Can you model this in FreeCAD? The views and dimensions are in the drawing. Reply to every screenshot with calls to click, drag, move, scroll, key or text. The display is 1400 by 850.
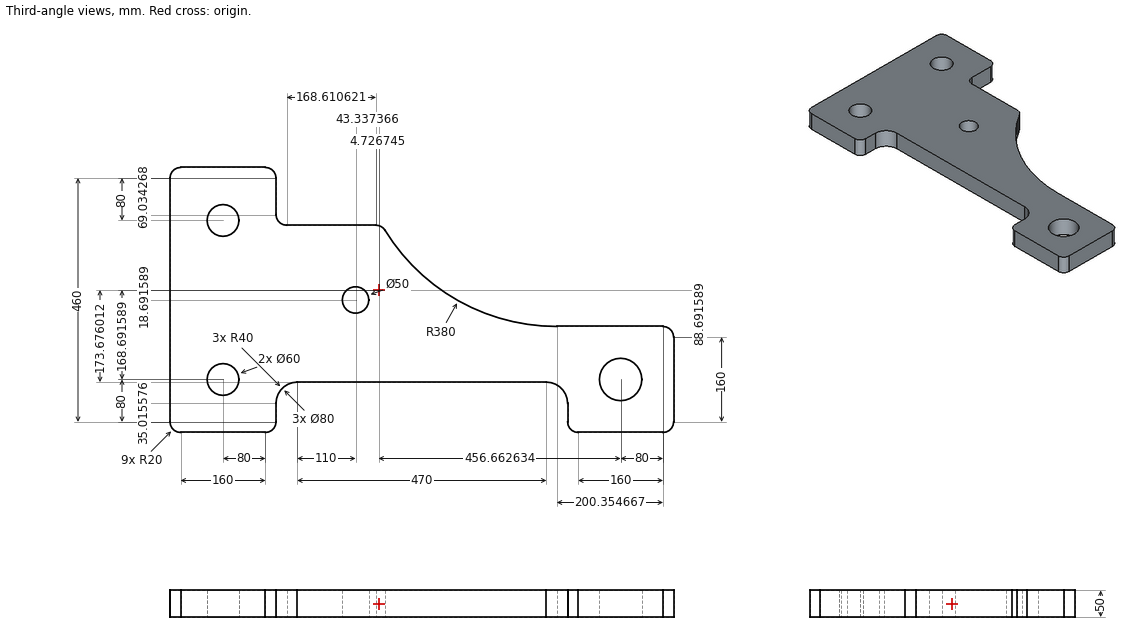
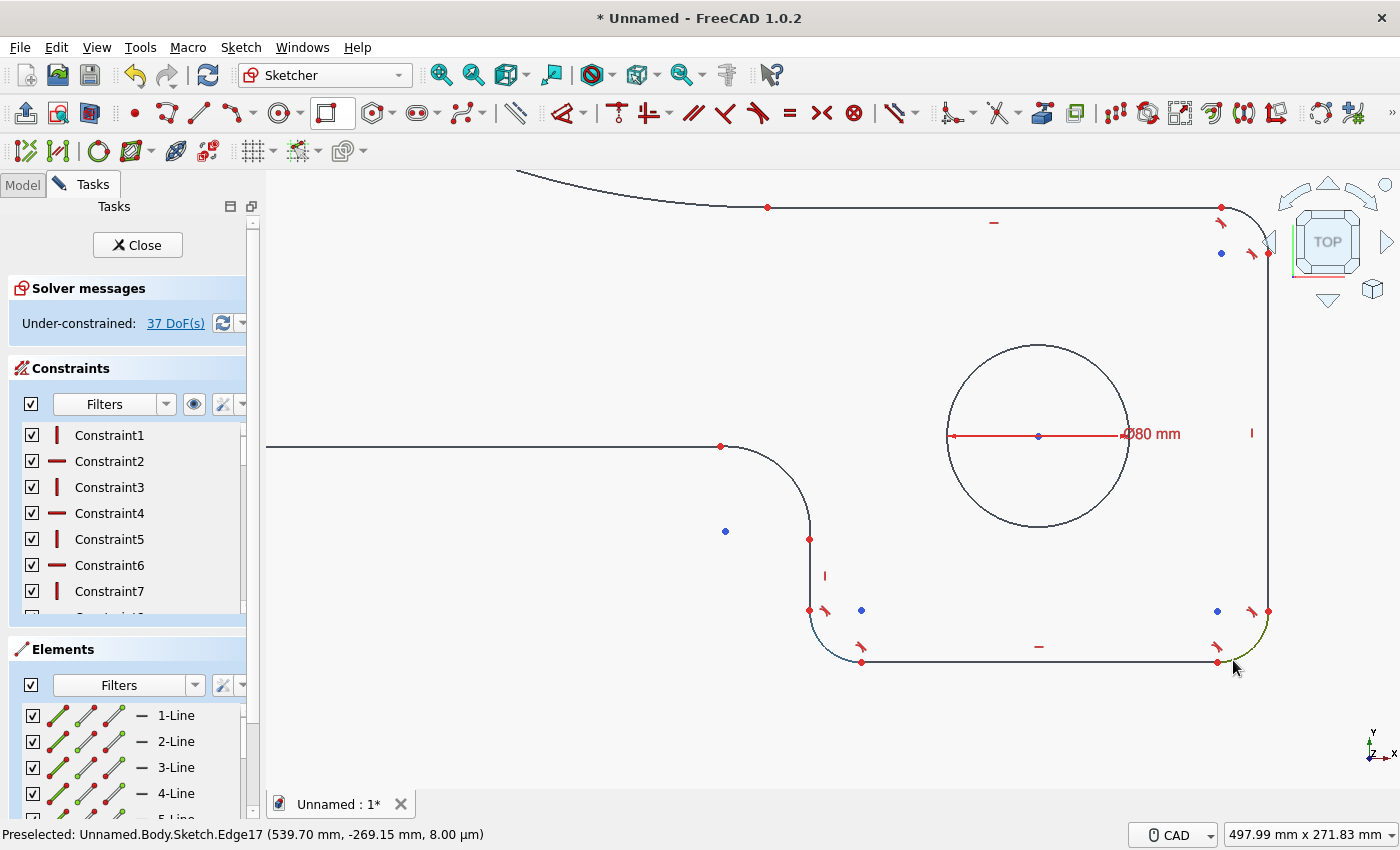
scroll(1014, 647, down, 6)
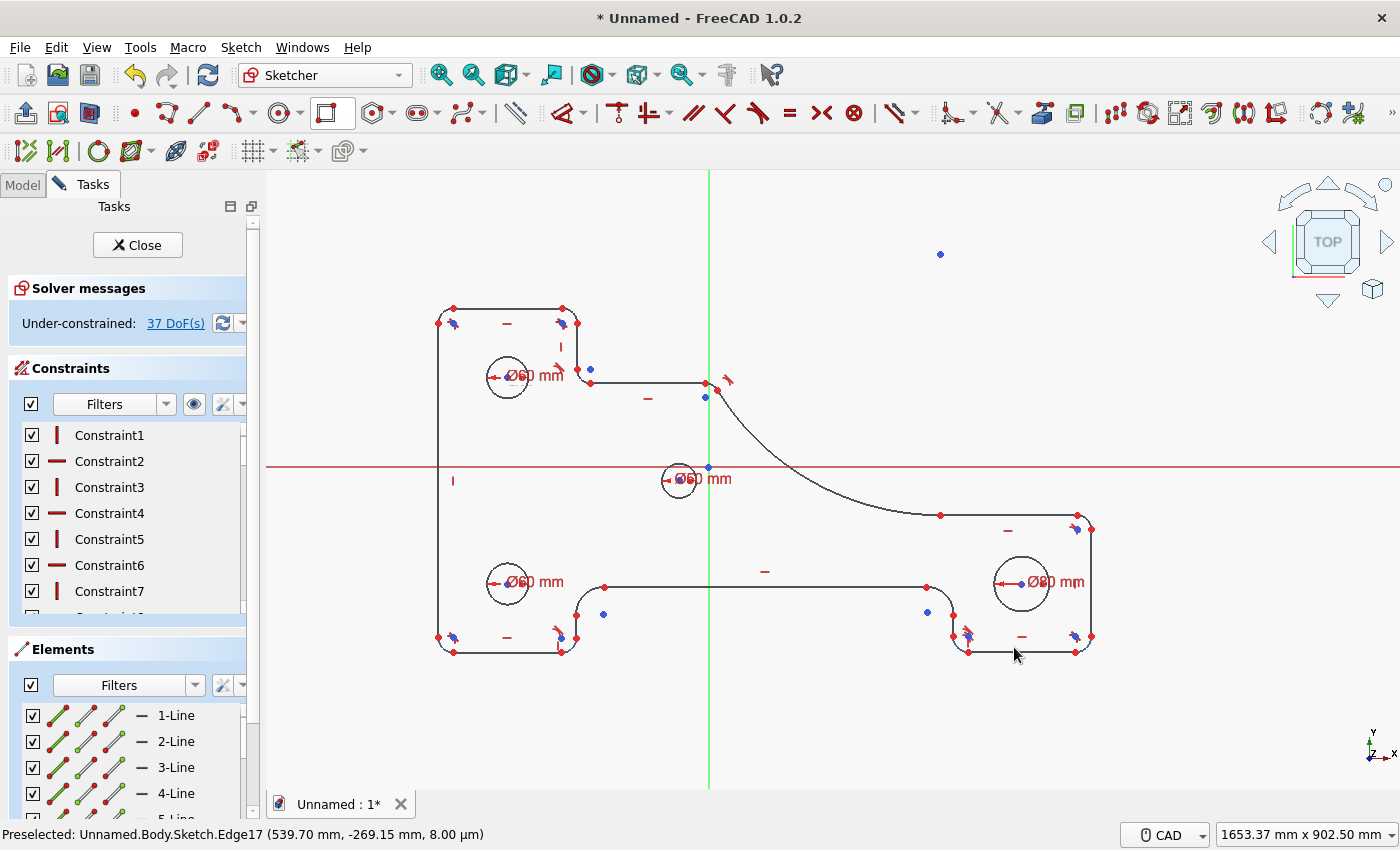
scroll(1090, 523, up, 4)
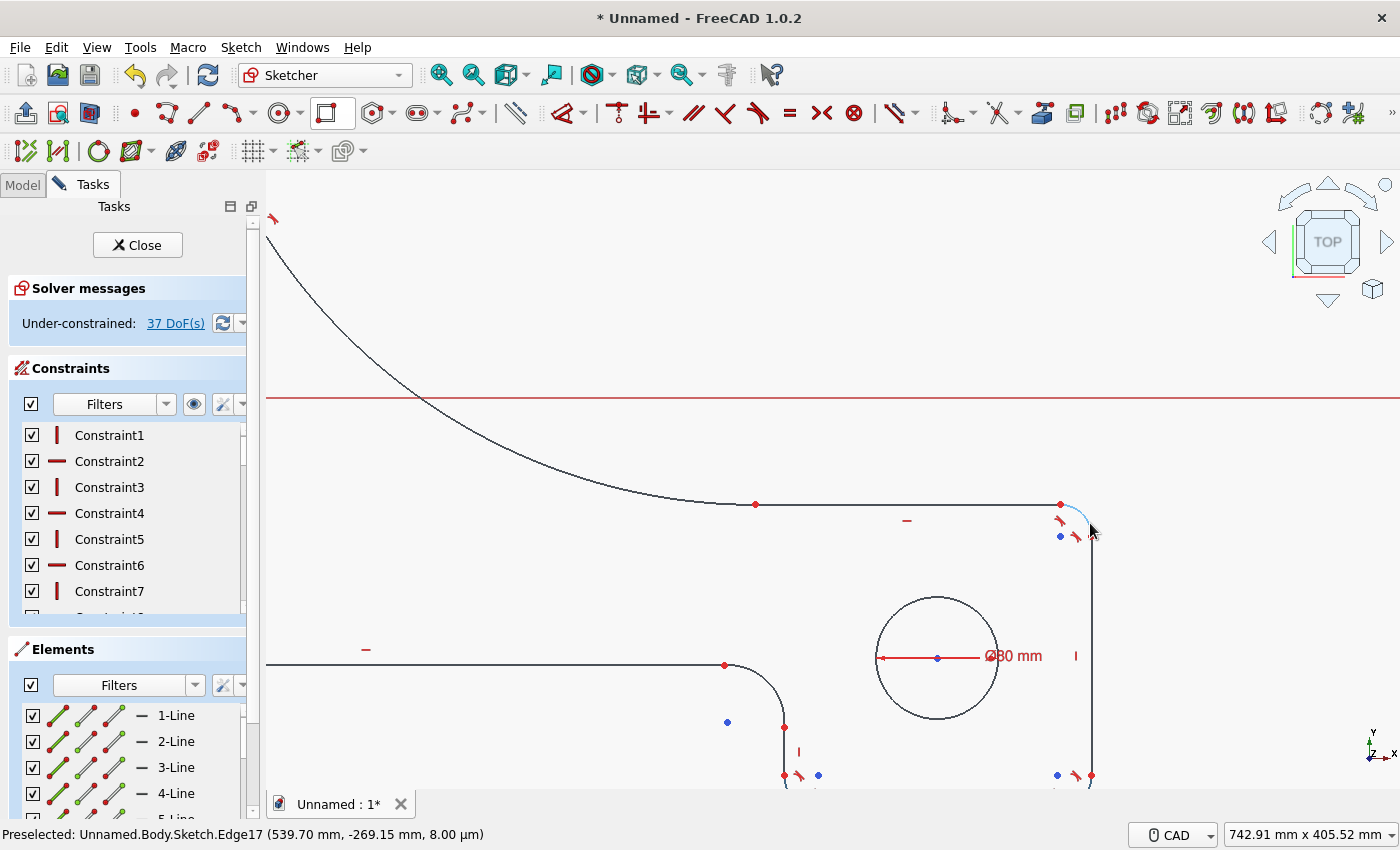
click(1088, 522)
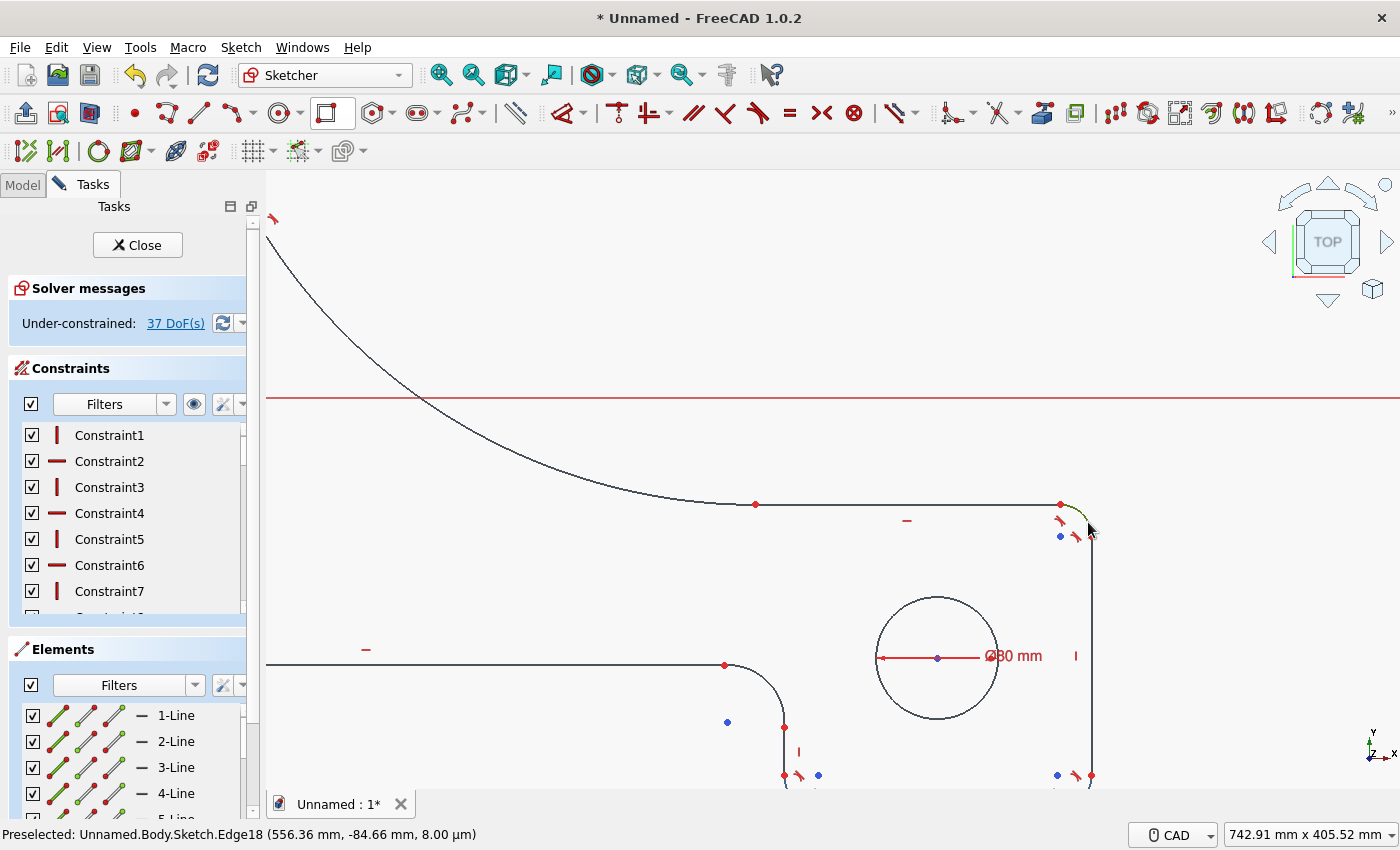
scroll(1090, 523, down, 4)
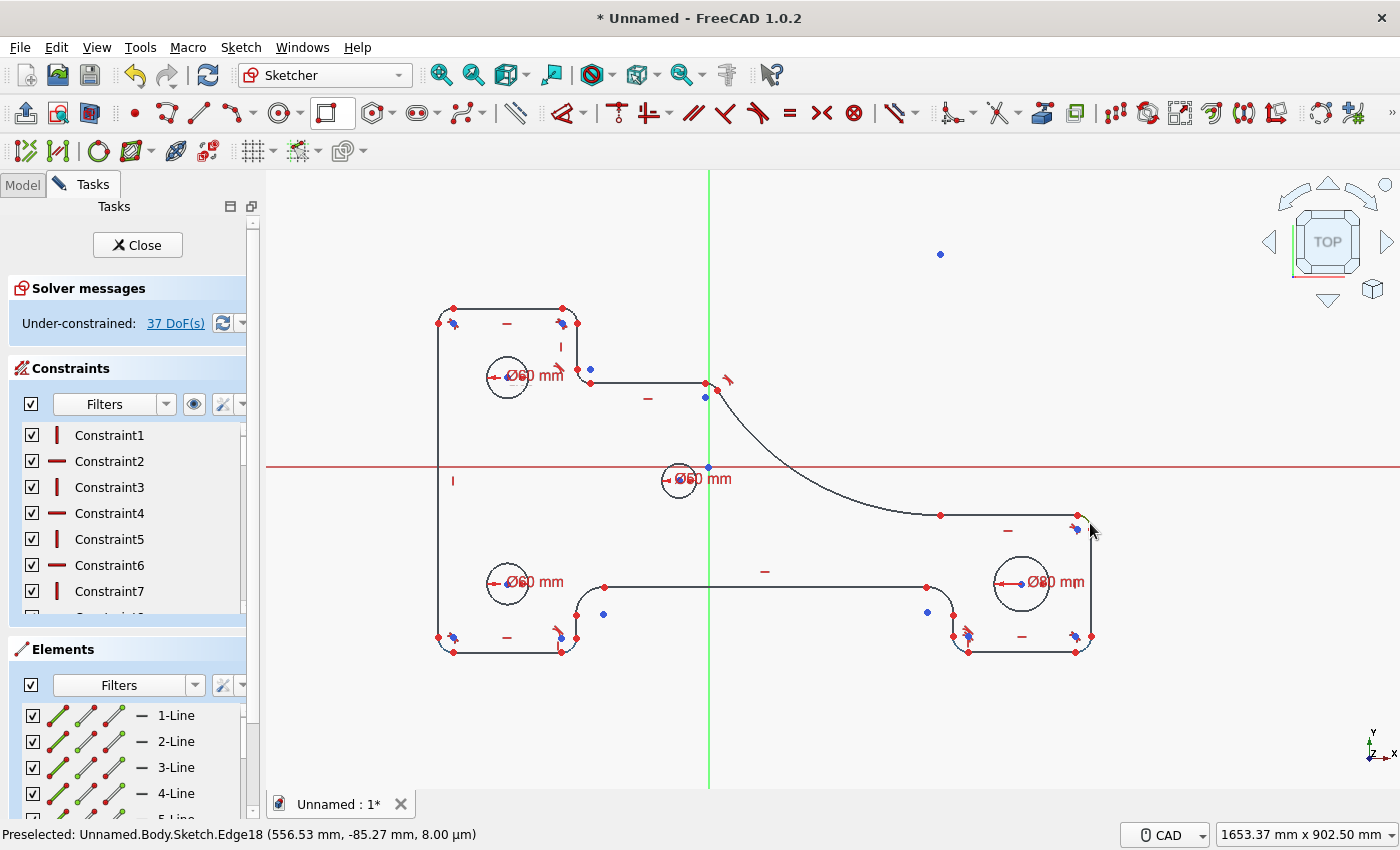
scroll(715, 387, up, 6)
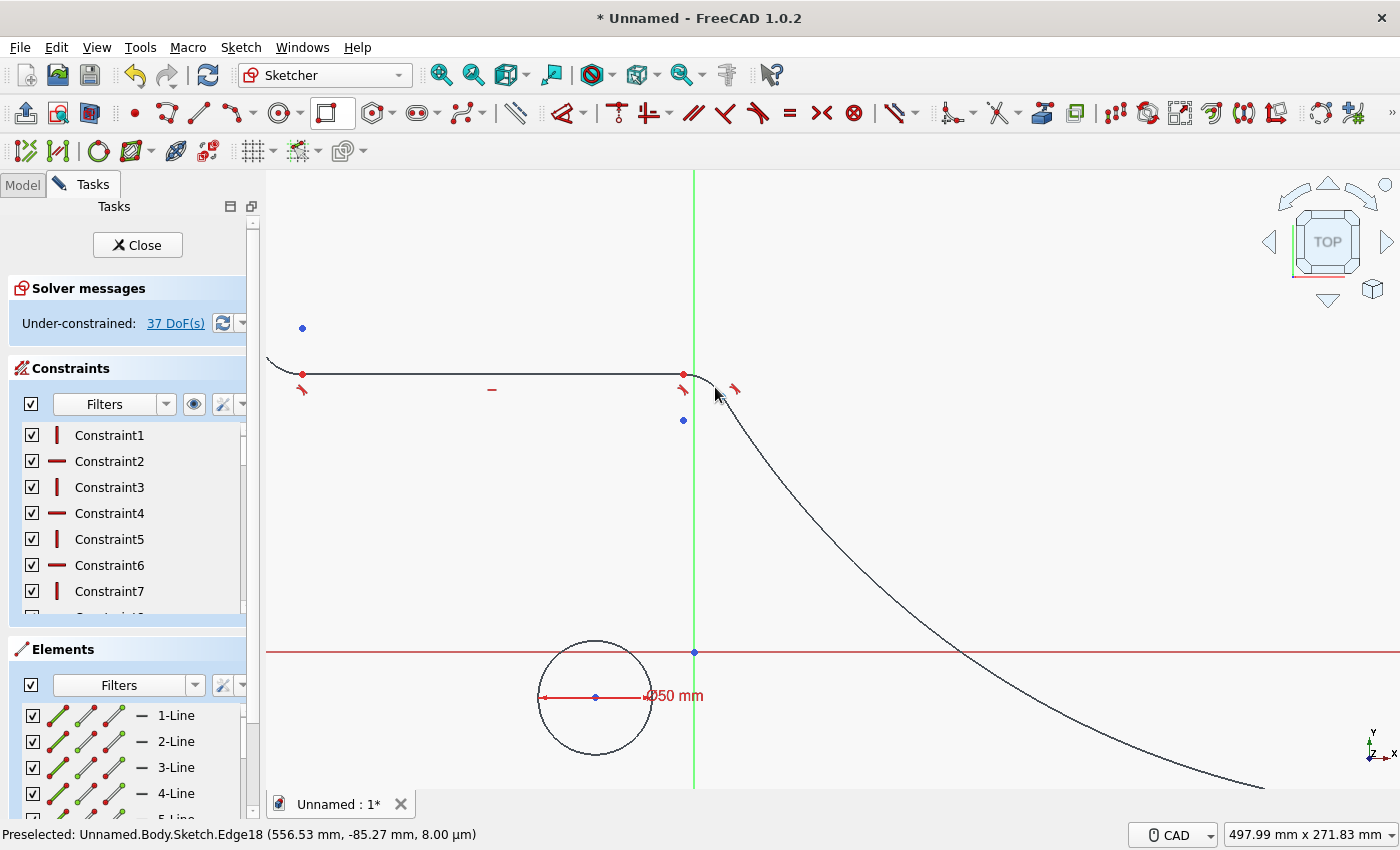
click(713, 386)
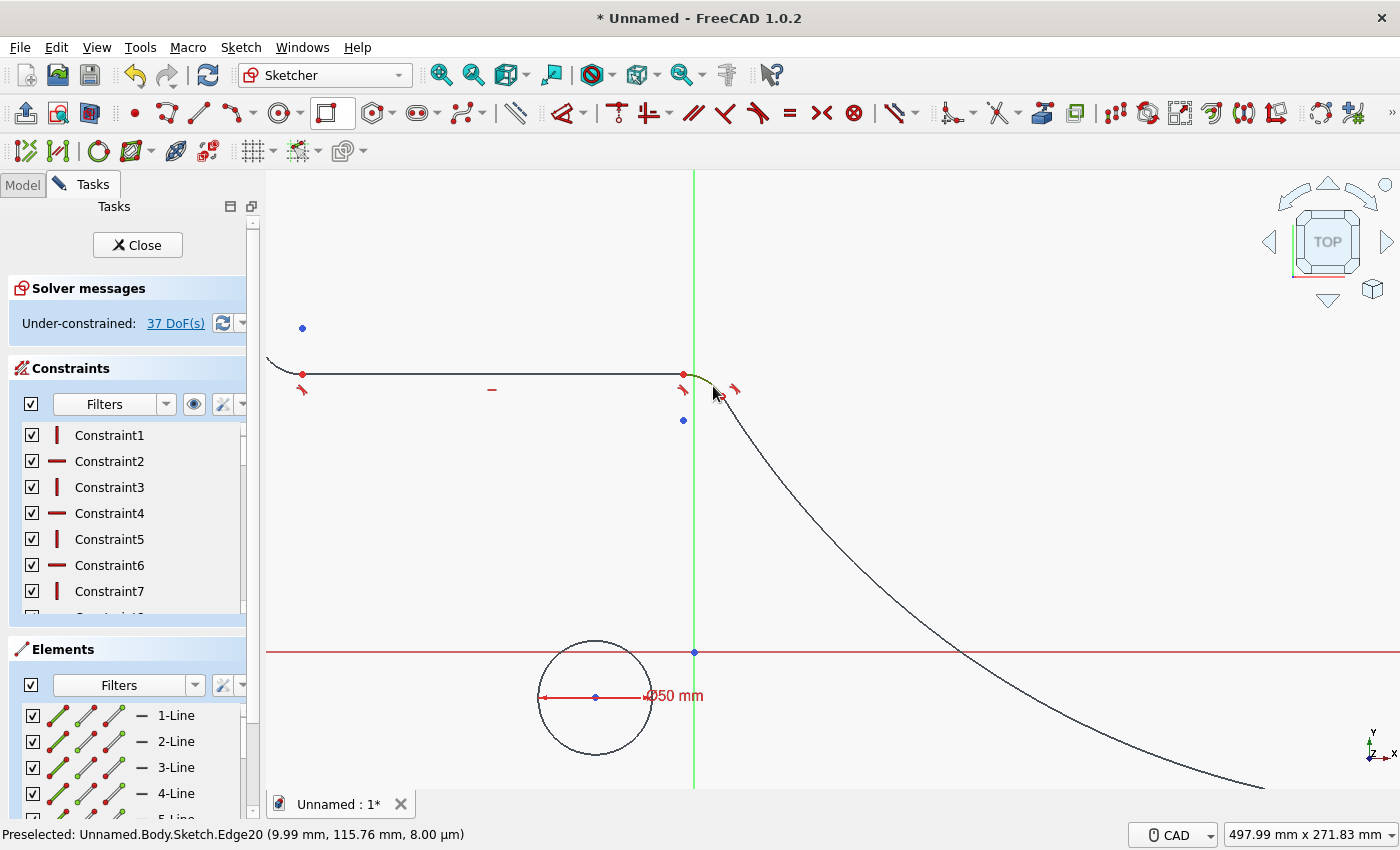
scroll(715, 387, down, 6)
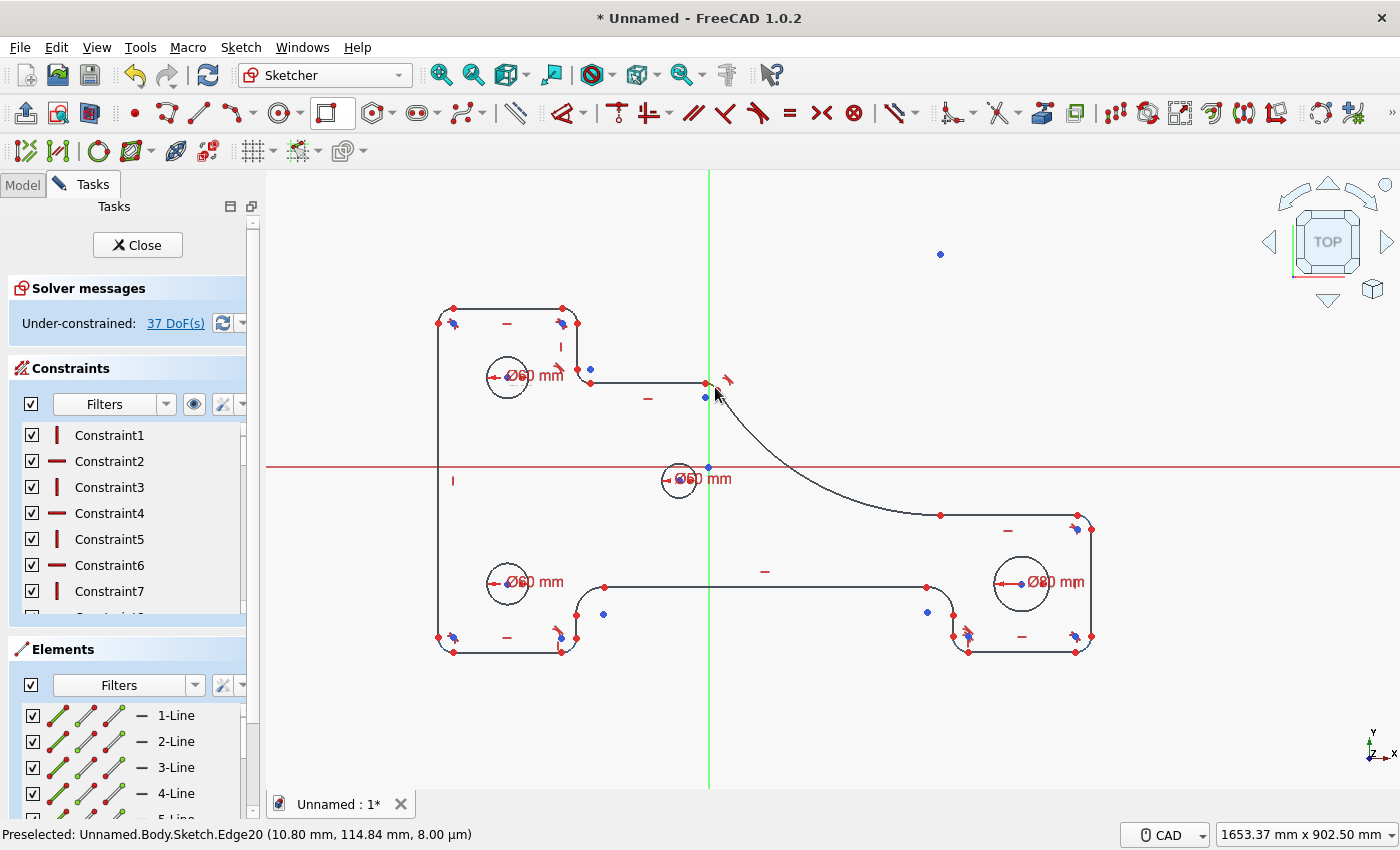
scroll(579, 376, up, 4)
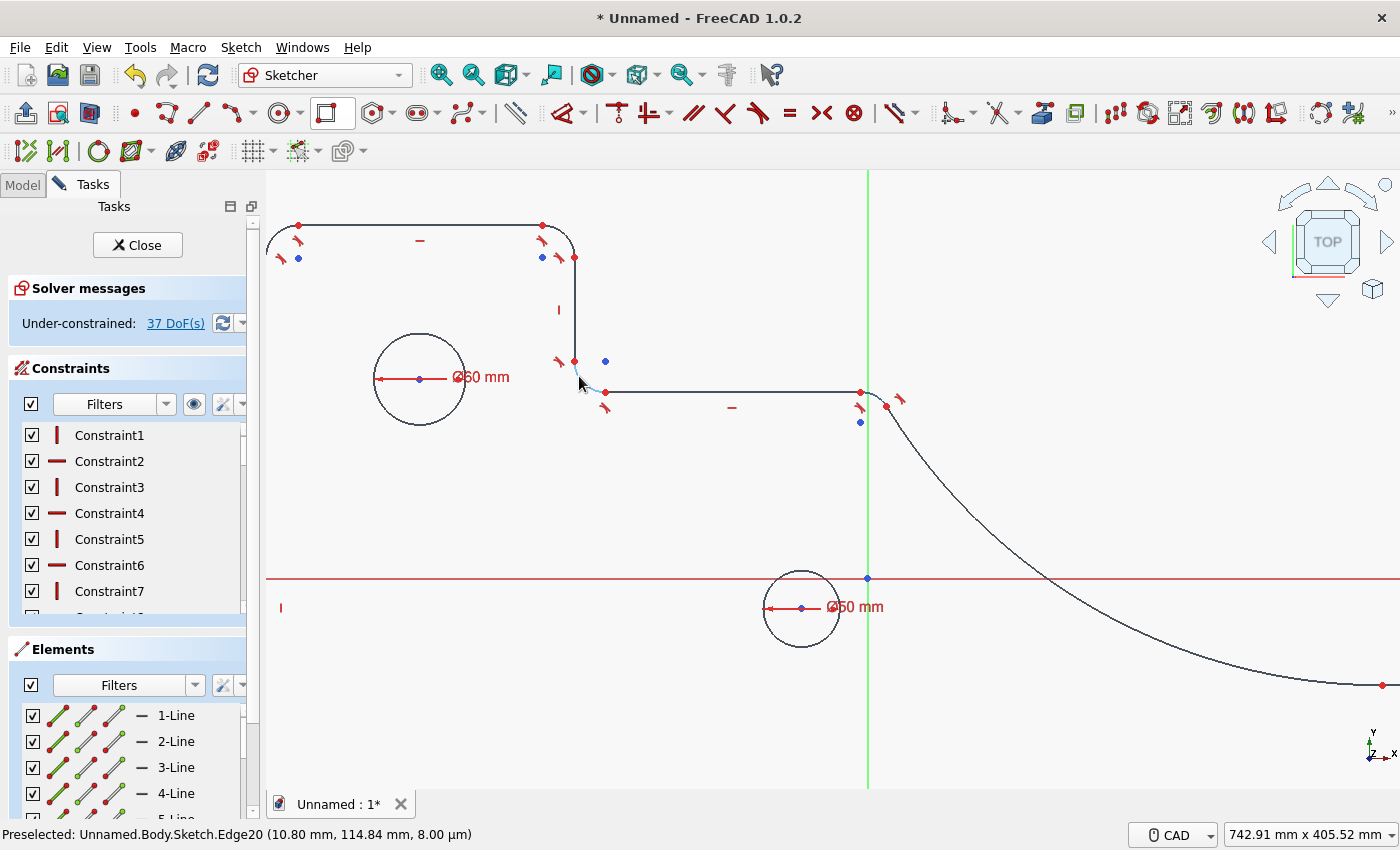
click(578, 375)